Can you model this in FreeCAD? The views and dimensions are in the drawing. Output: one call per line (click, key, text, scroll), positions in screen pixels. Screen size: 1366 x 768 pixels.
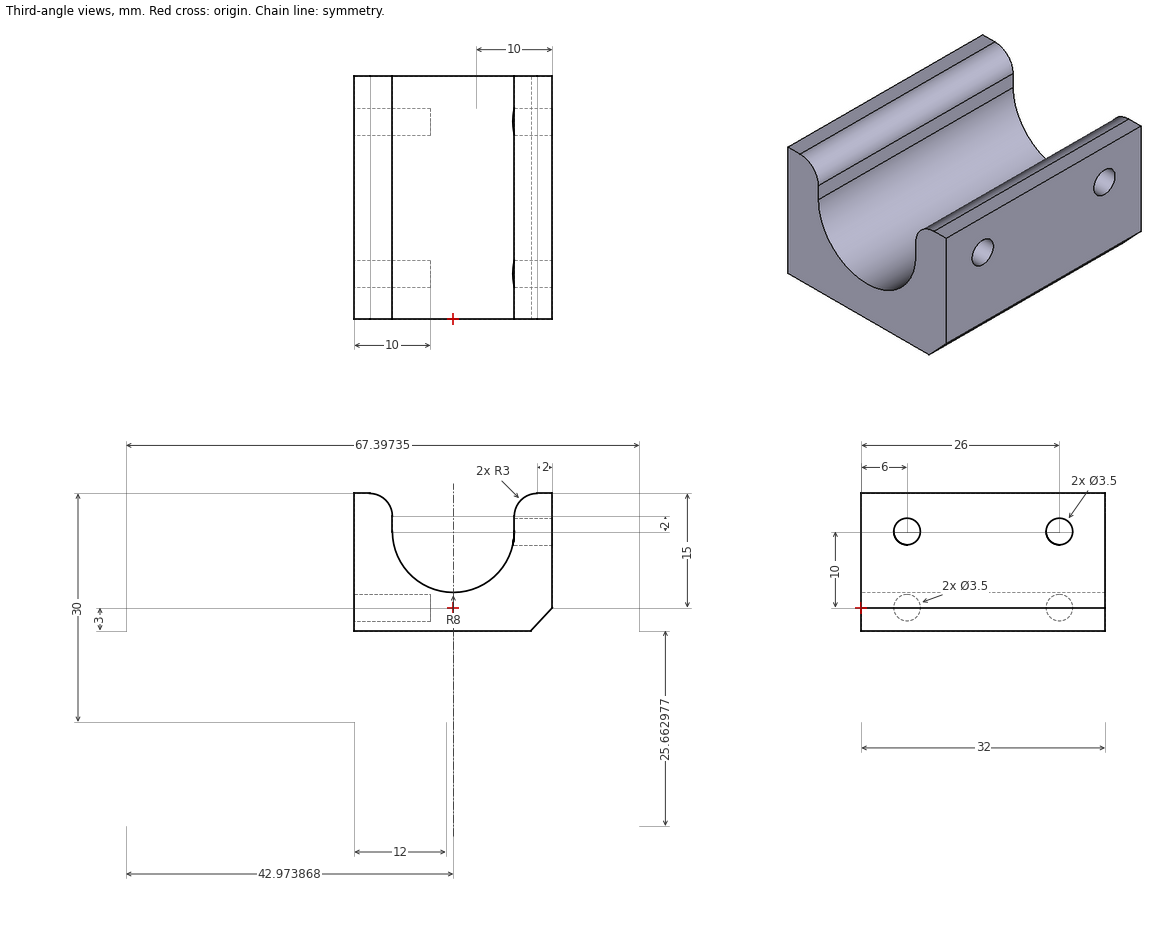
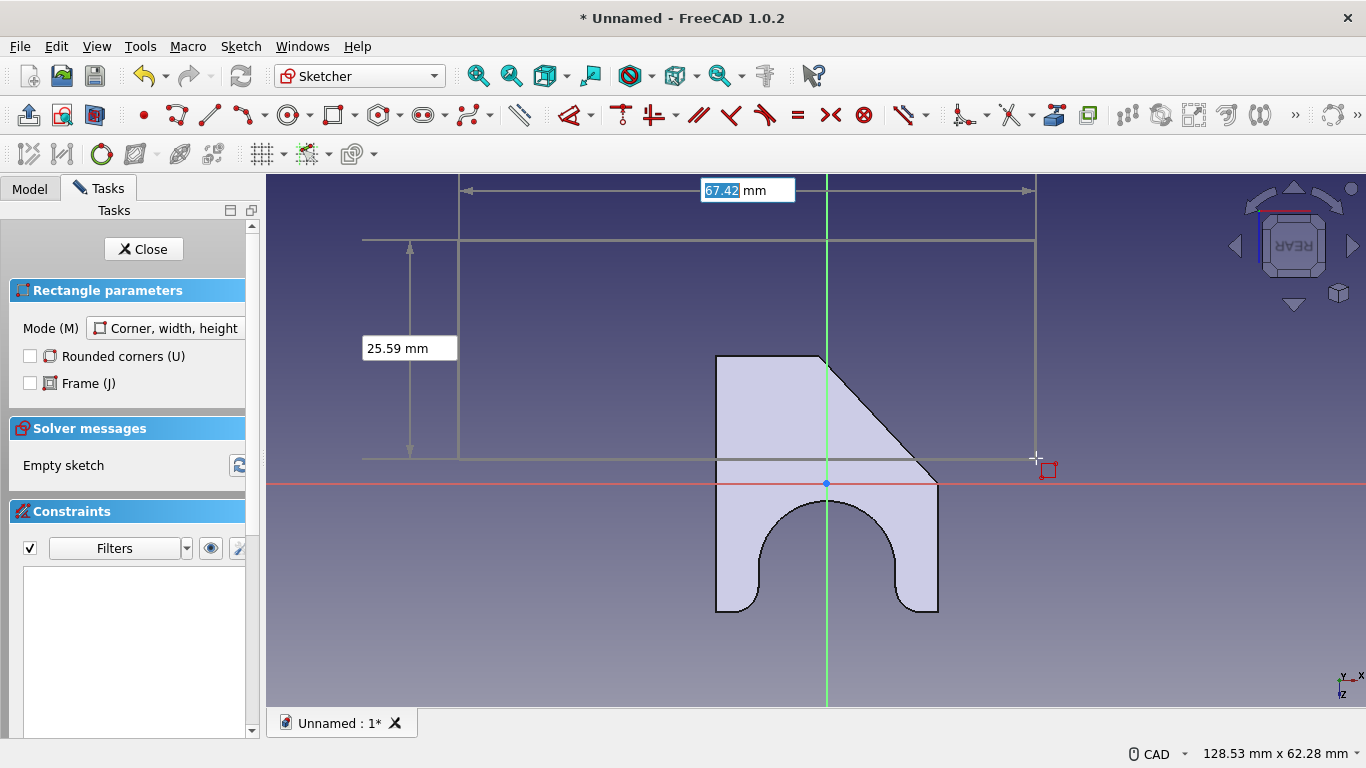
text(67.39735)
key(Tab)
text(25.662977)
key(Return)
key(Escape)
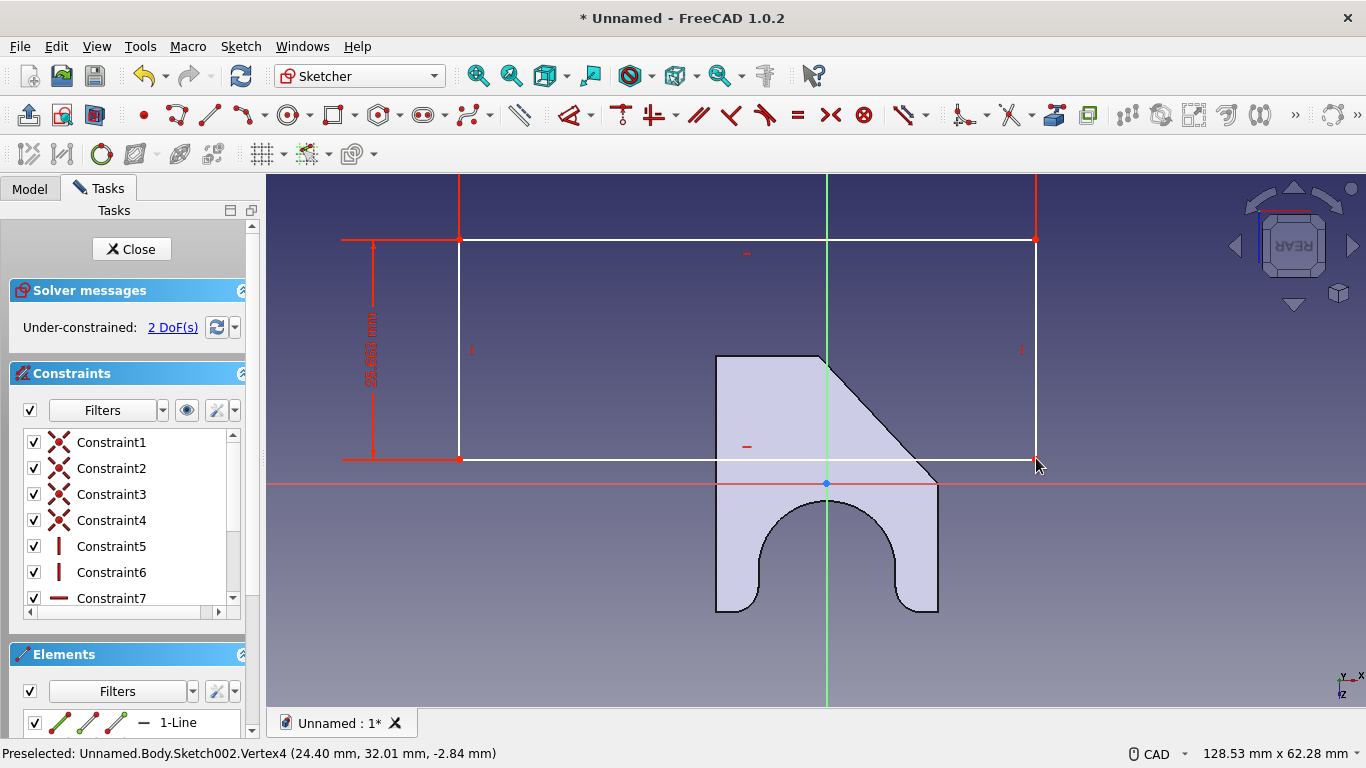
click(568, 116)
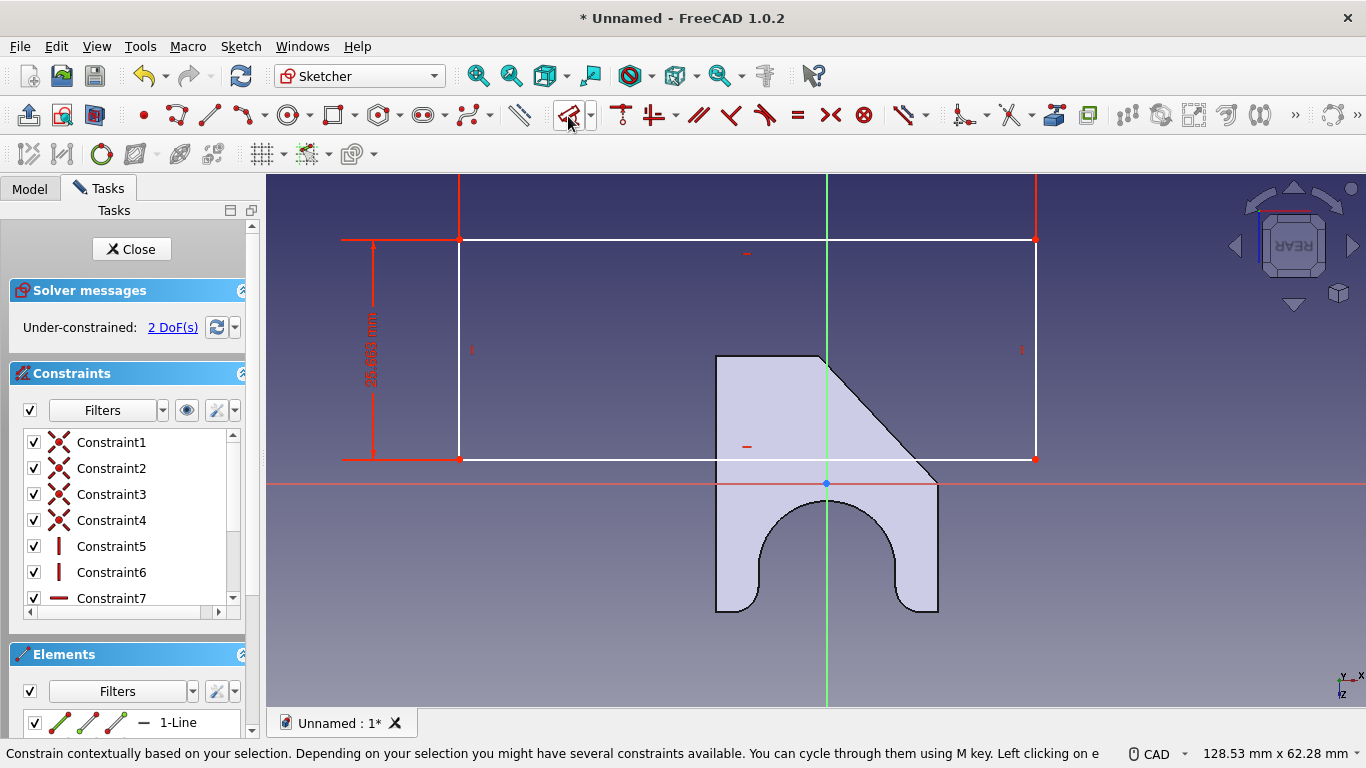
scroll(459, 460, up, 3)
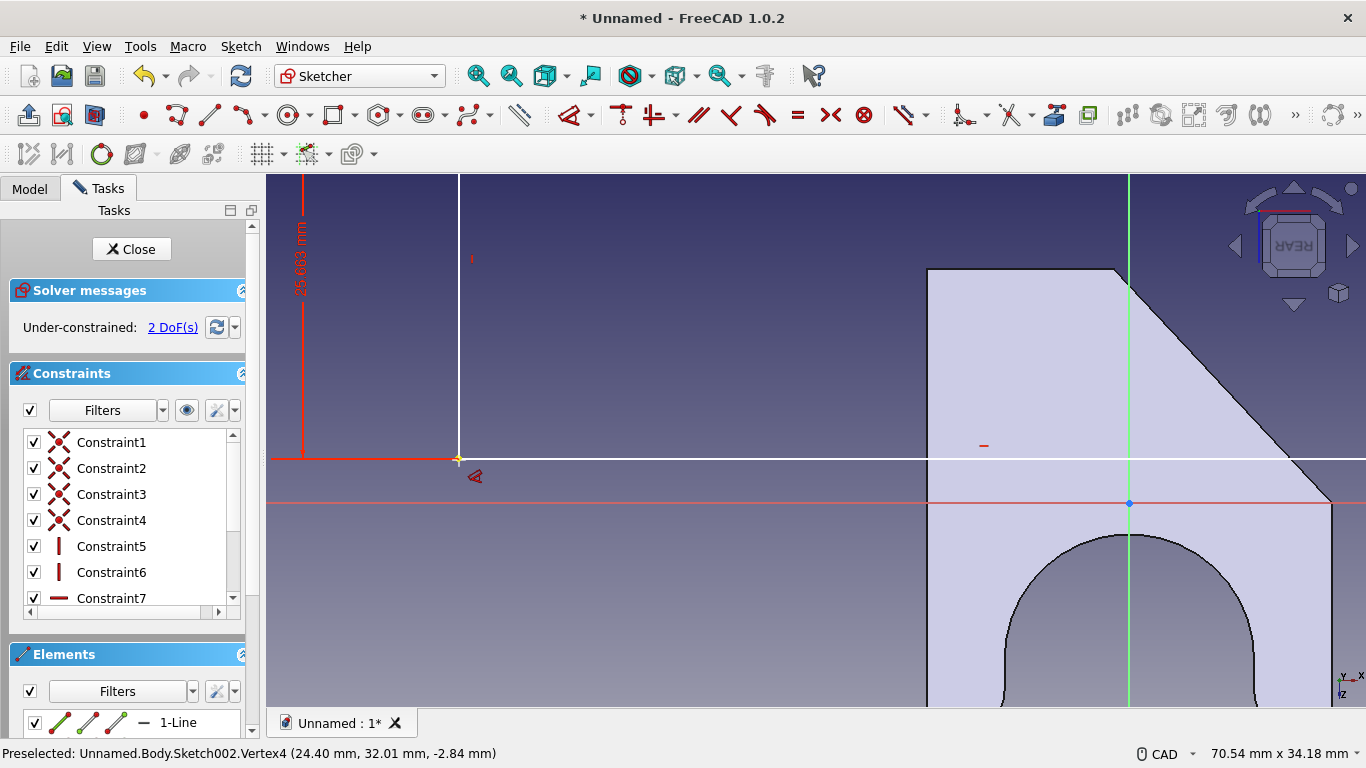
click(459, 459)
click(425, 481)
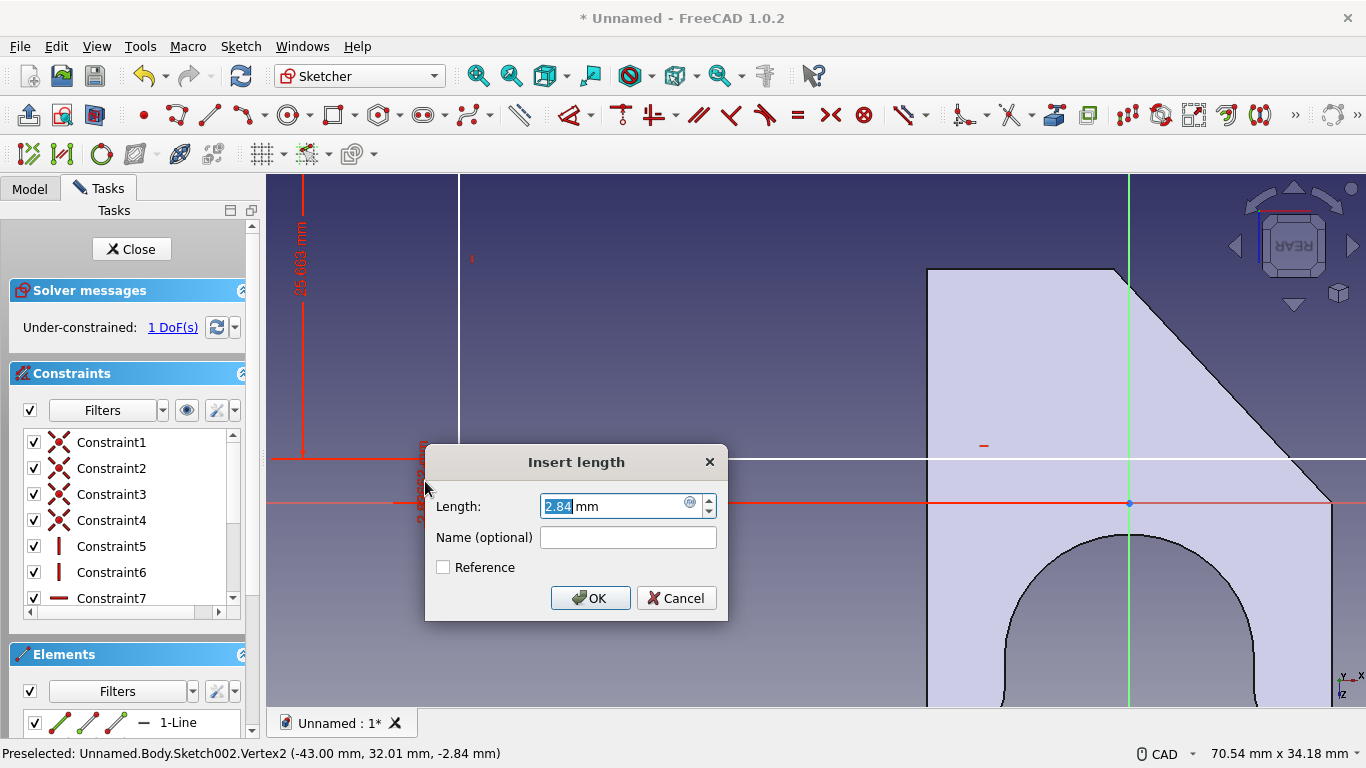
text(3)
key(Return)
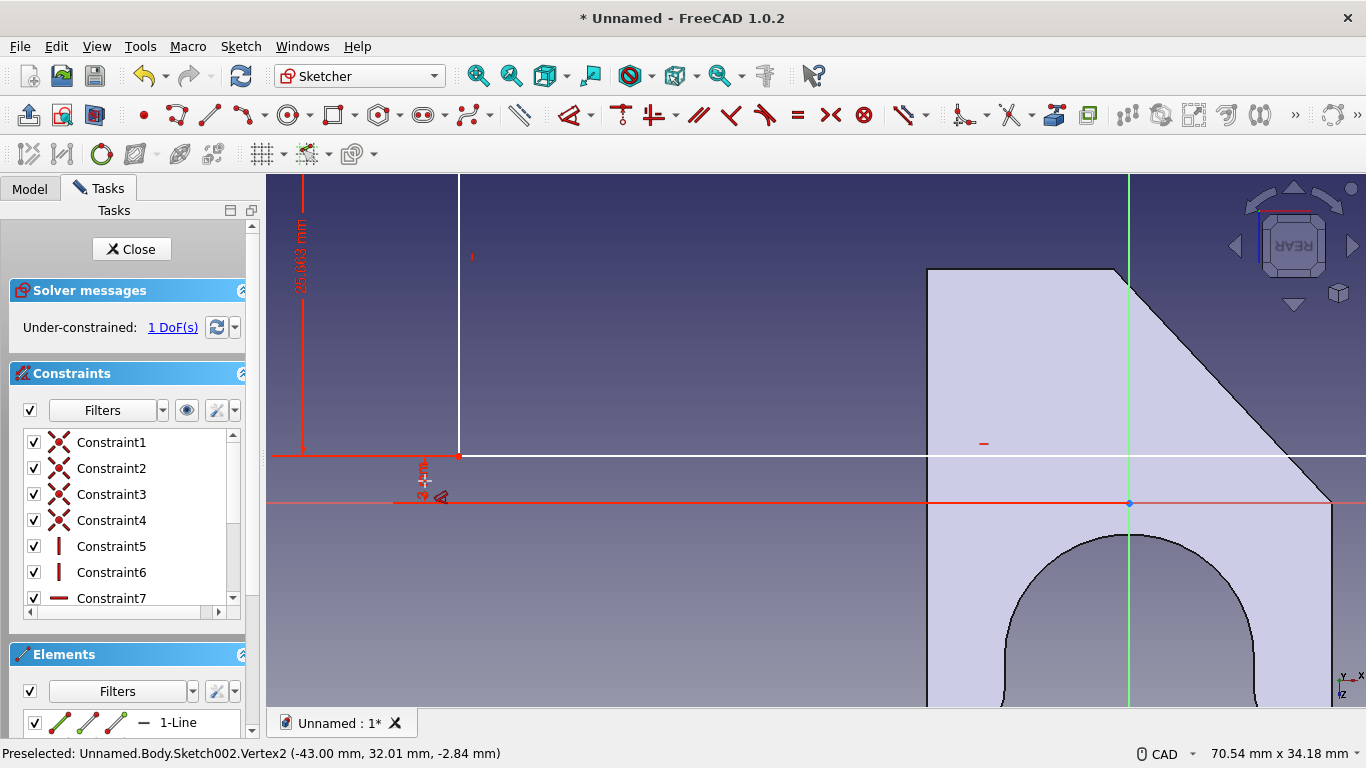
scroll(294, 679, down, 2)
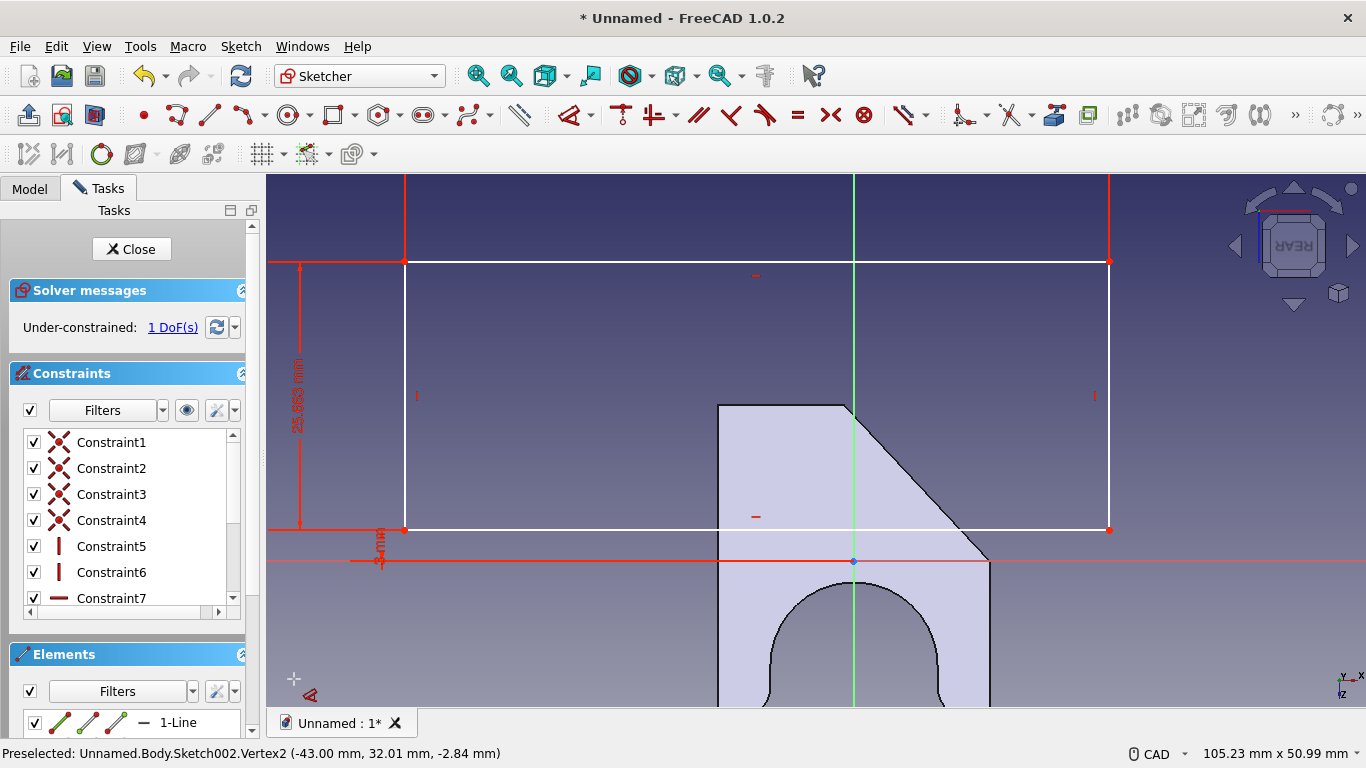
click(405, 262)
click(629, 228)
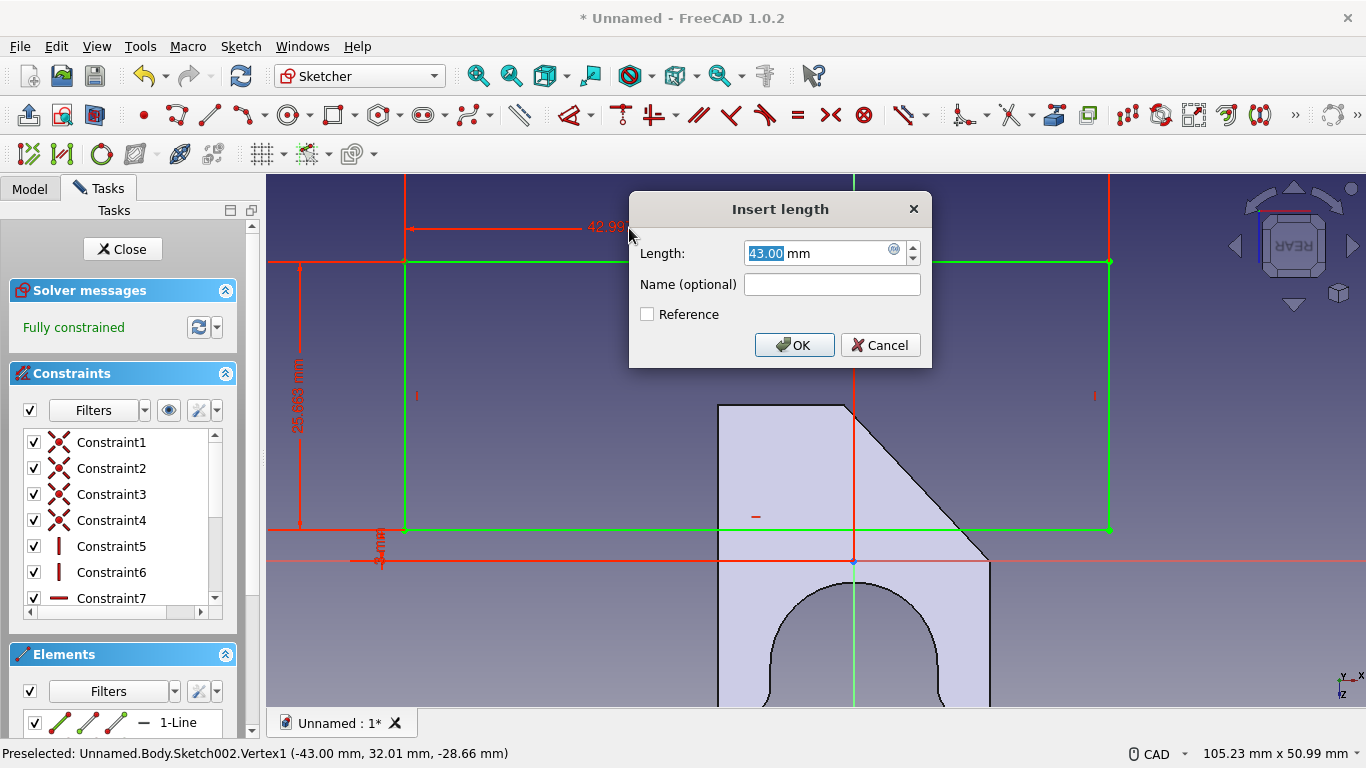
text(42.973868)
key(Return)
key(Escape)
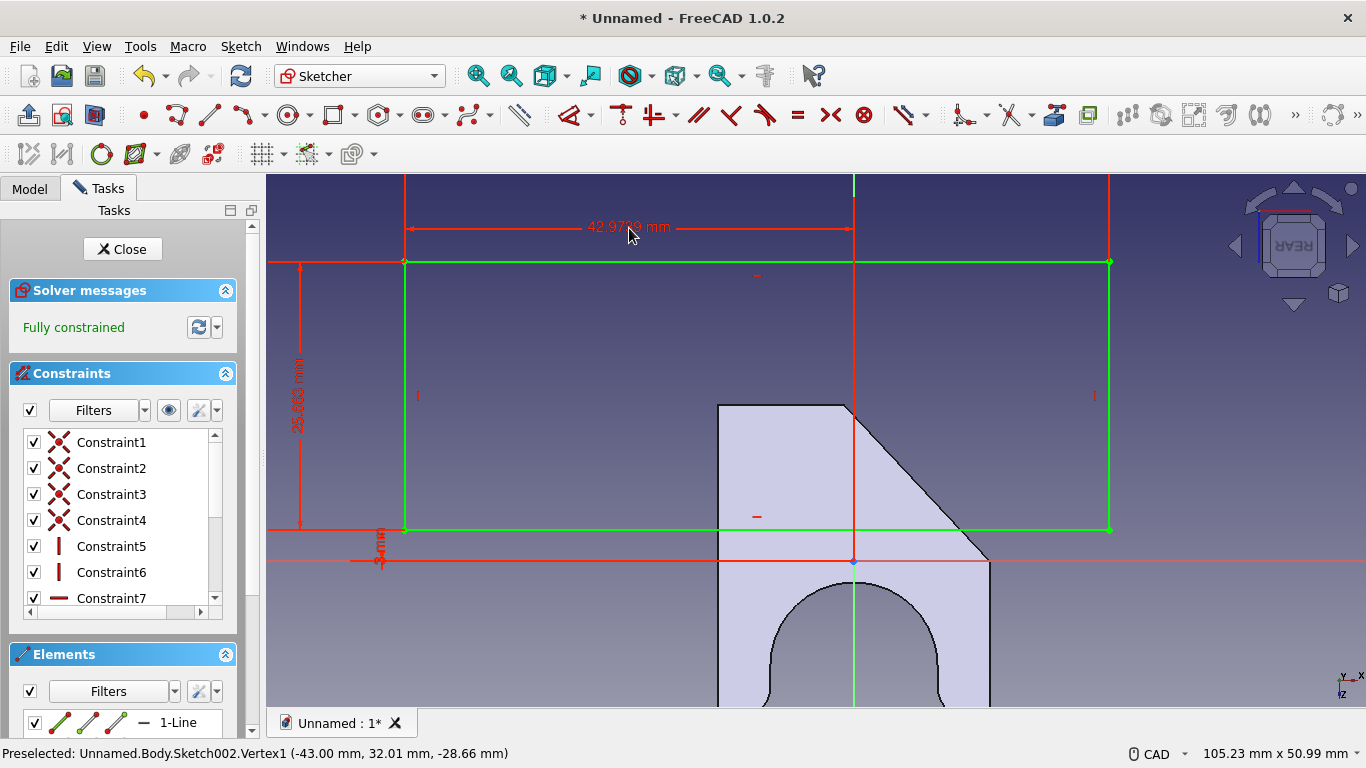
click(123, 249)